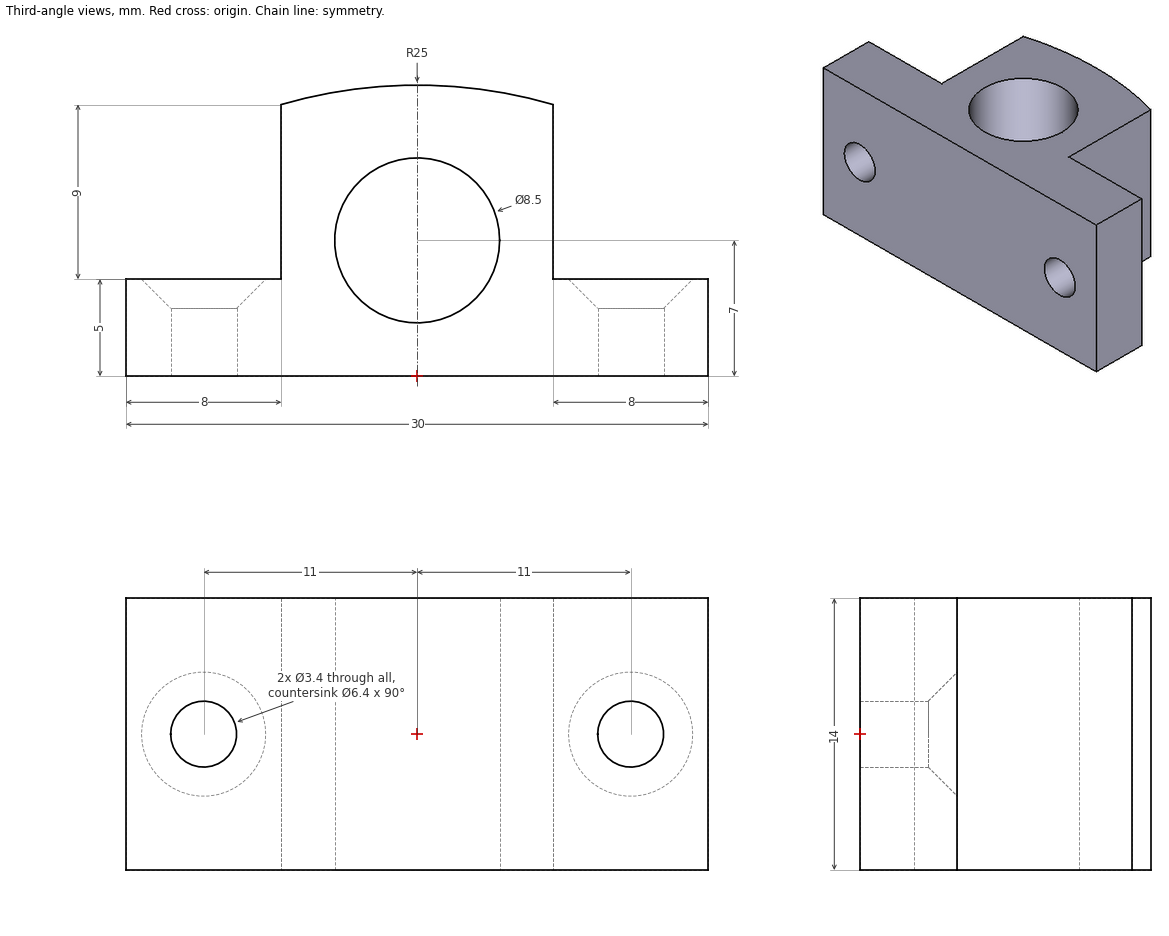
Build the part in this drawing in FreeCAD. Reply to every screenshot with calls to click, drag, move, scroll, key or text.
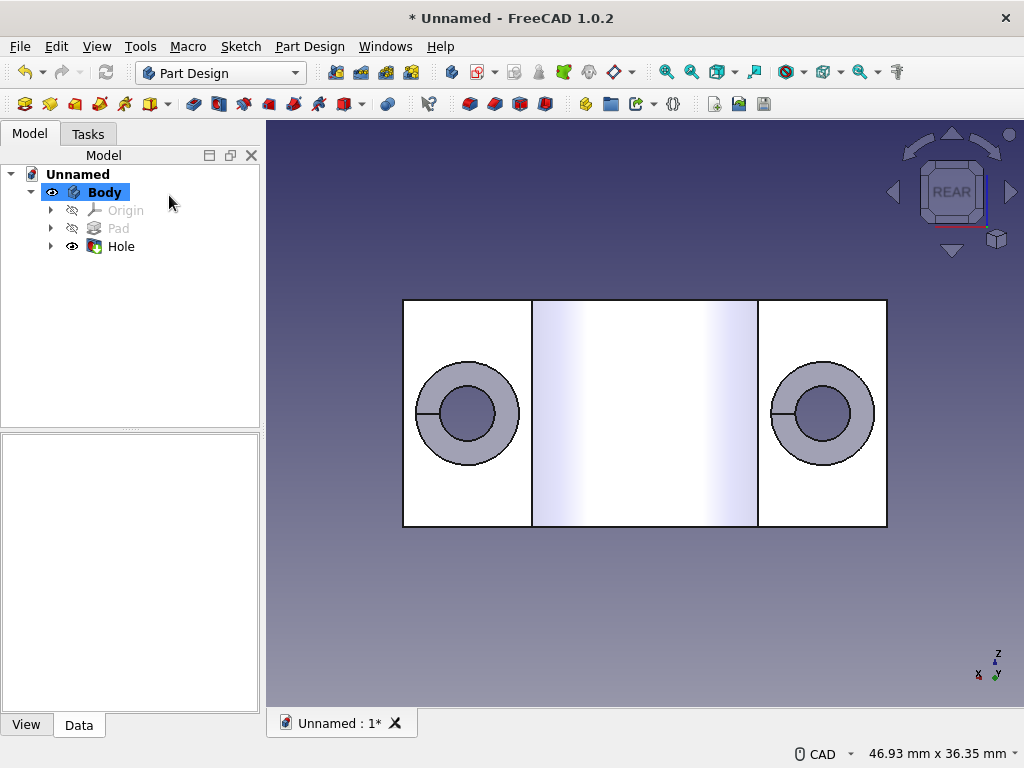
key(0)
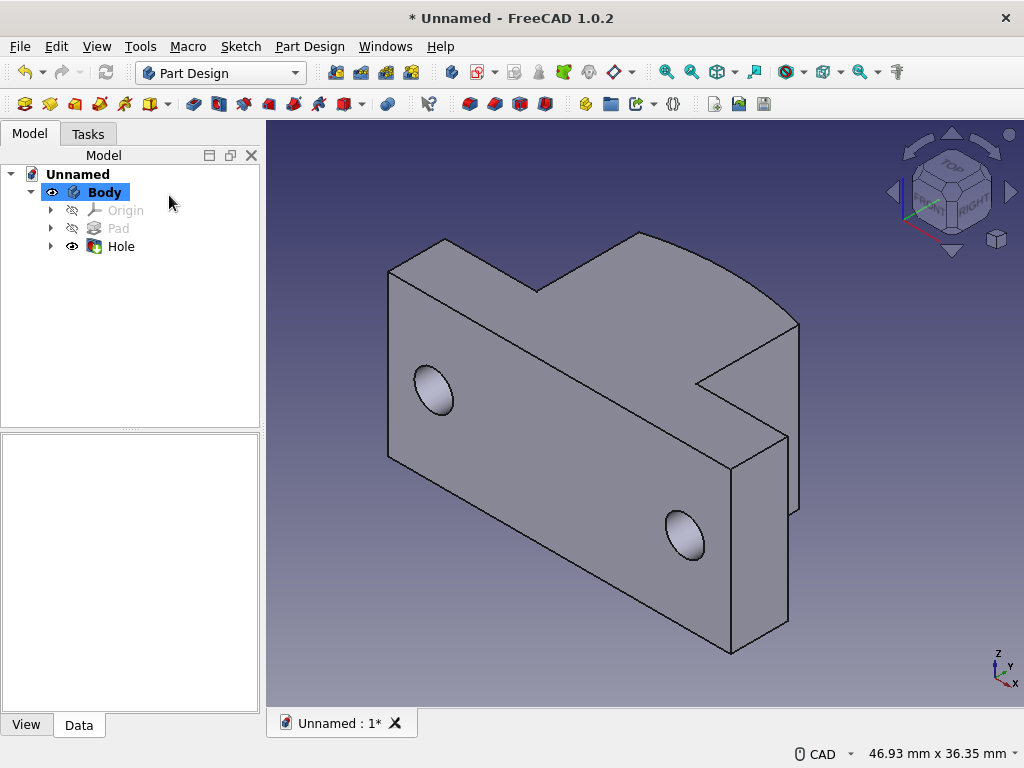
click(645, 320)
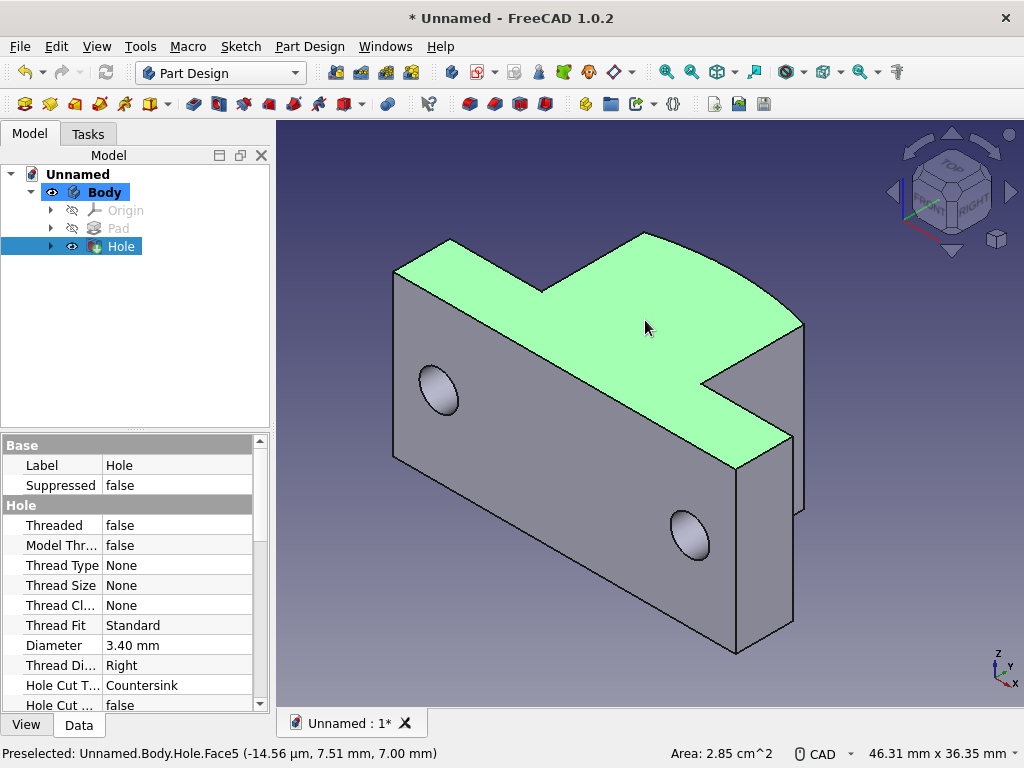
click(476, 72)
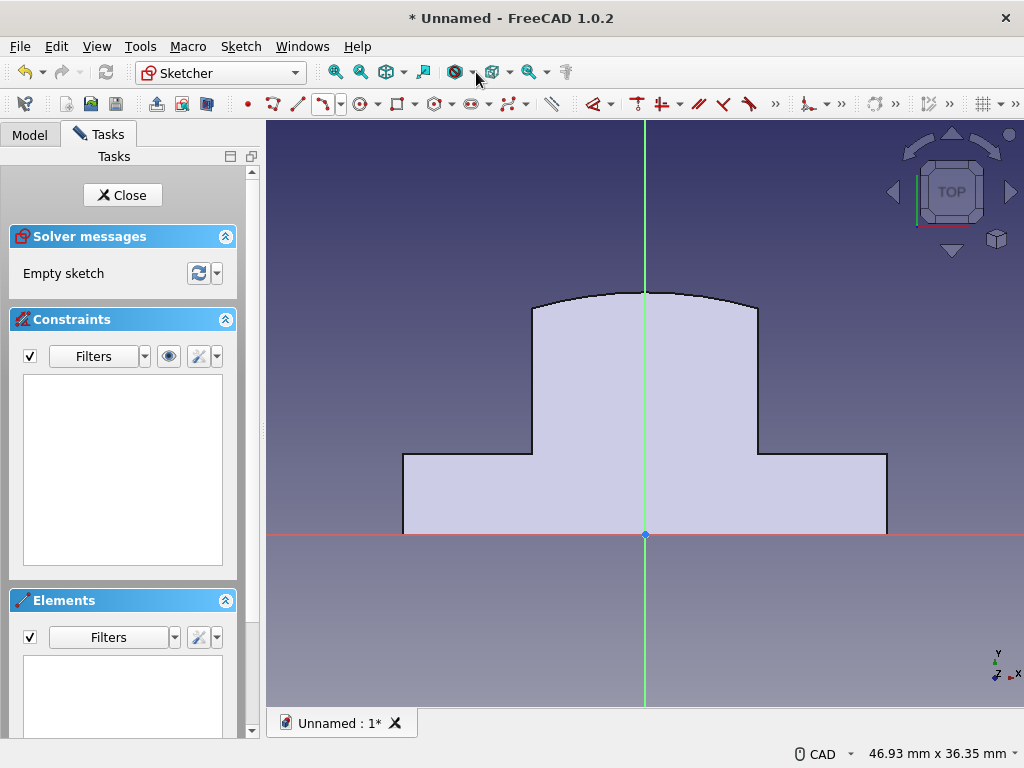
scroll(701, 468, up, 4)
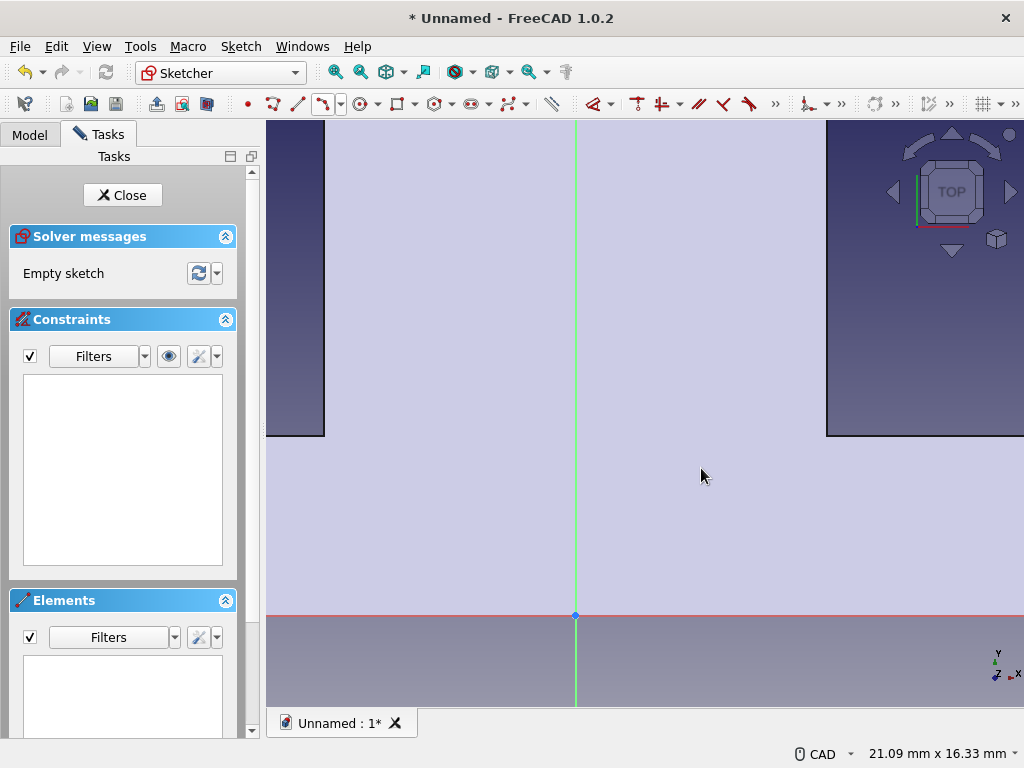
click(360, 104)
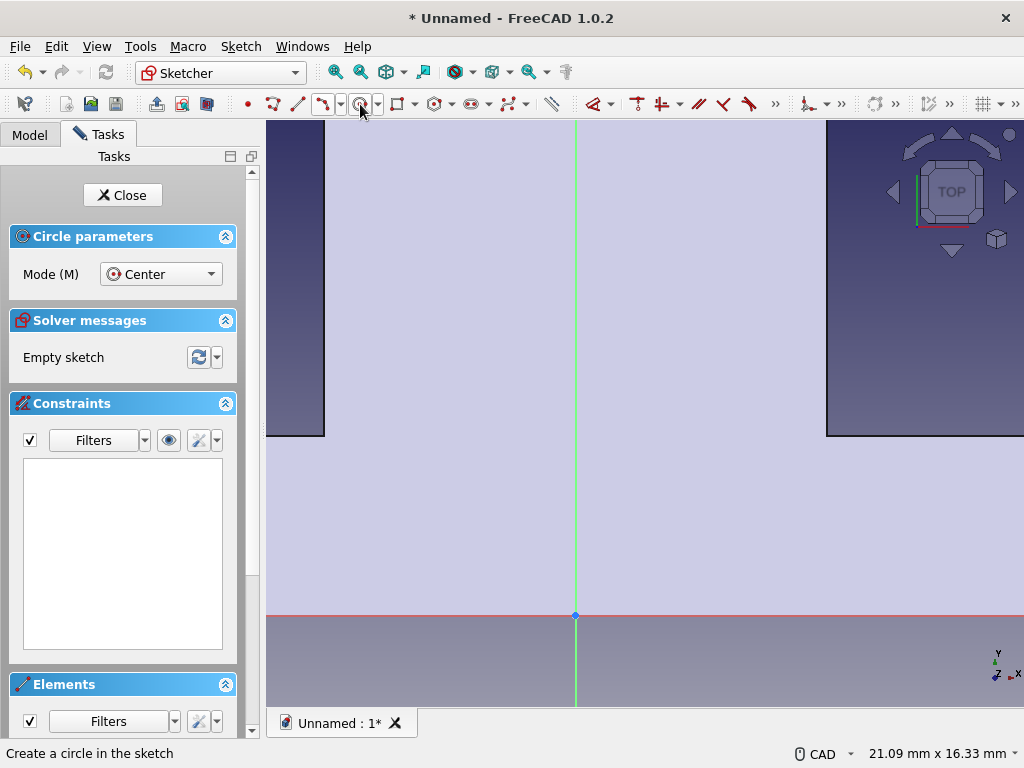
click(576, 364)
move(684, 256)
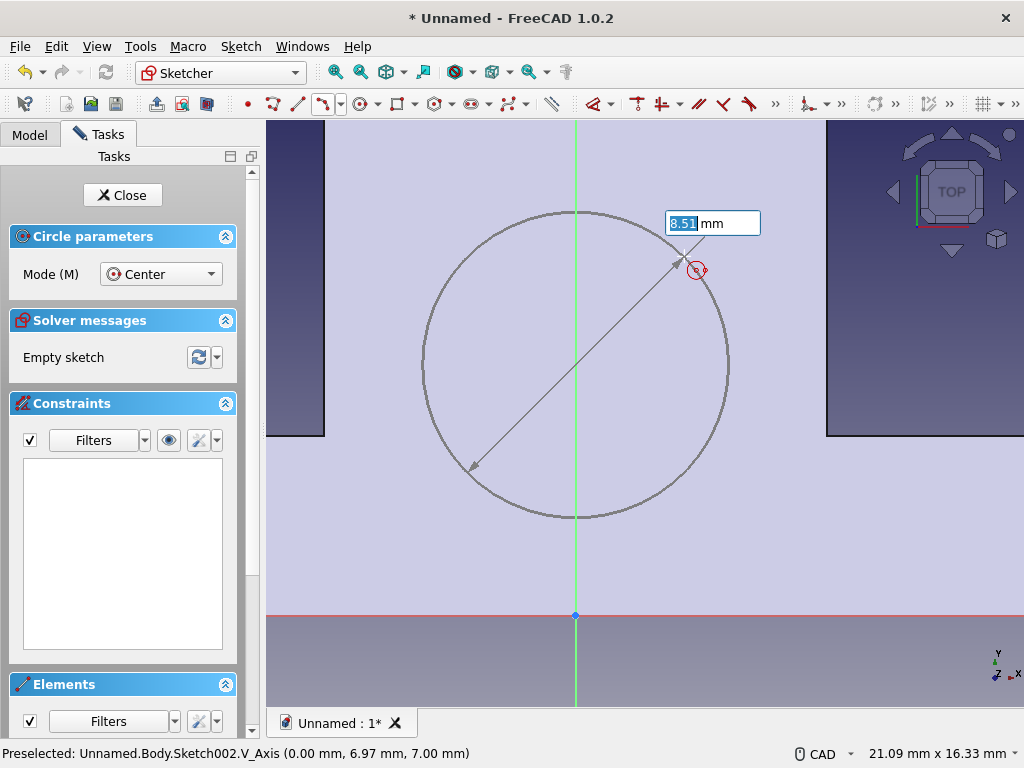
text(8.5)
key(Return)
key(Escape)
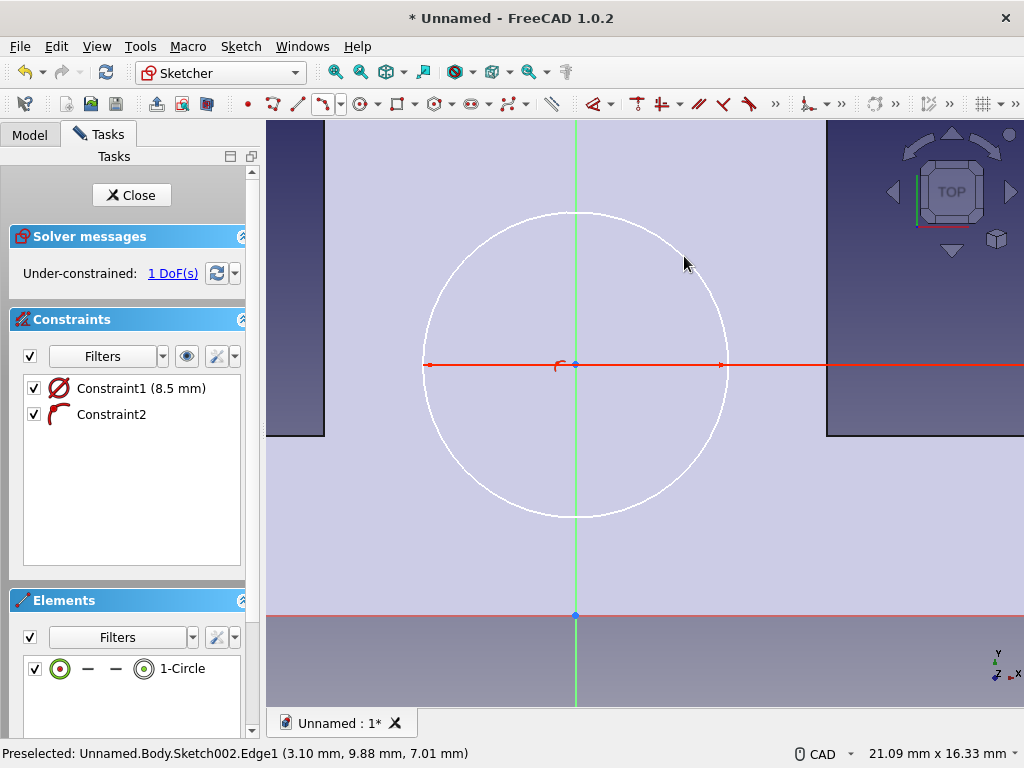
click(592, 104)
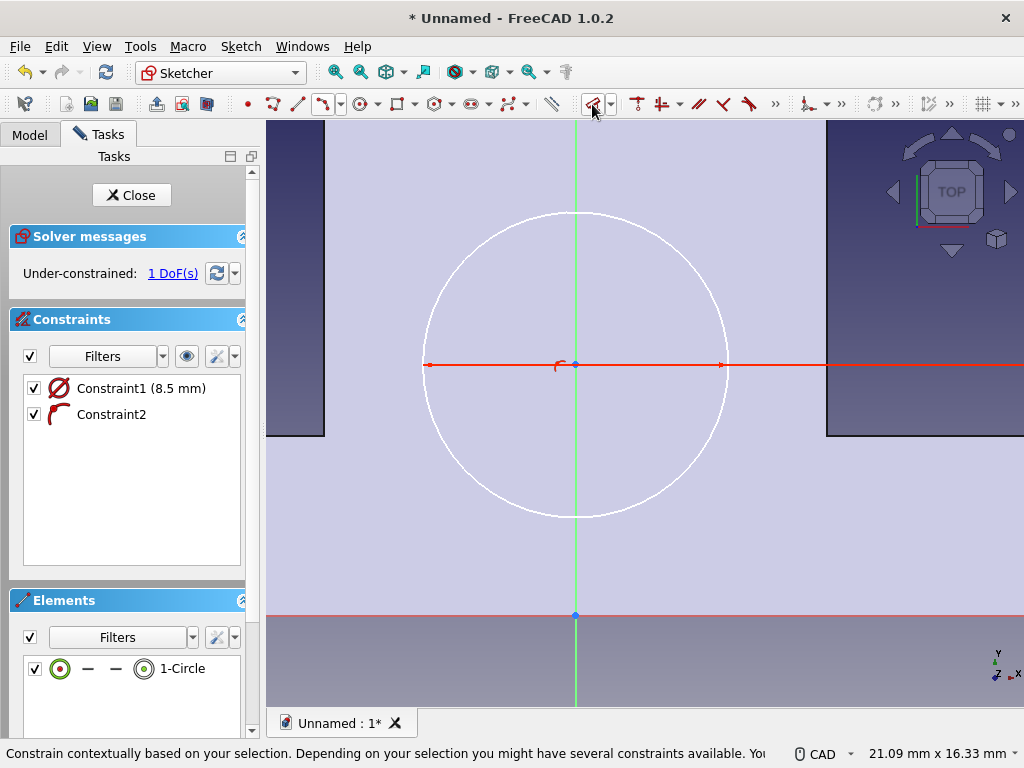
click(576, 365)
click(610, 490)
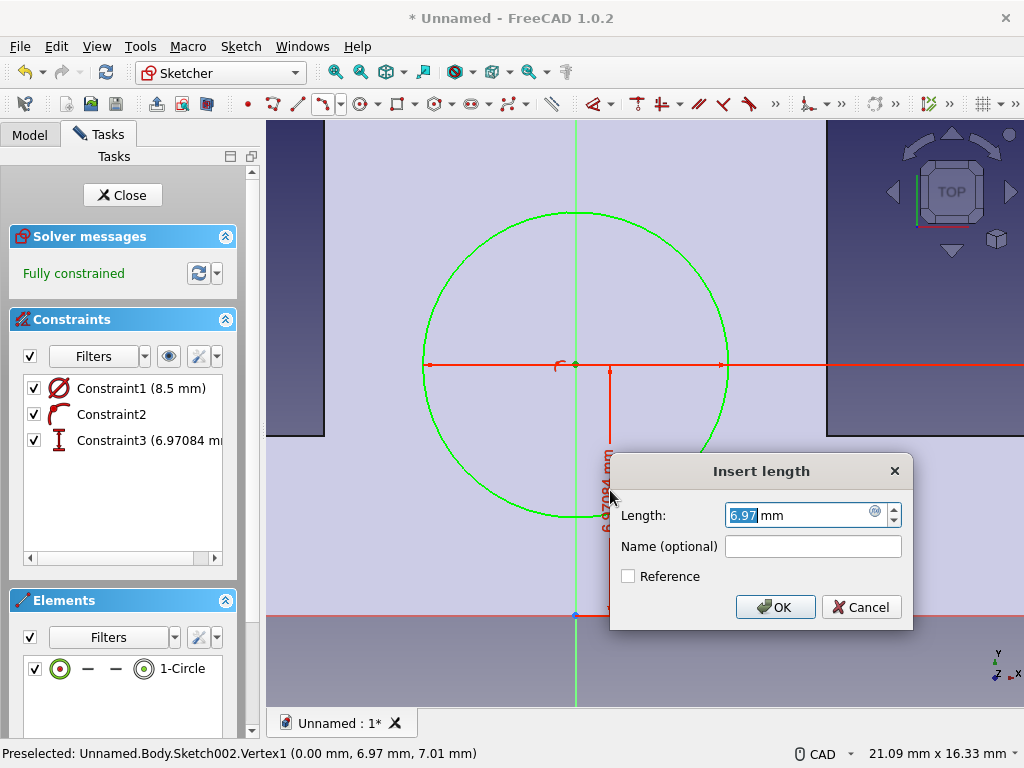
text(7)
key(Return)
key(Escape)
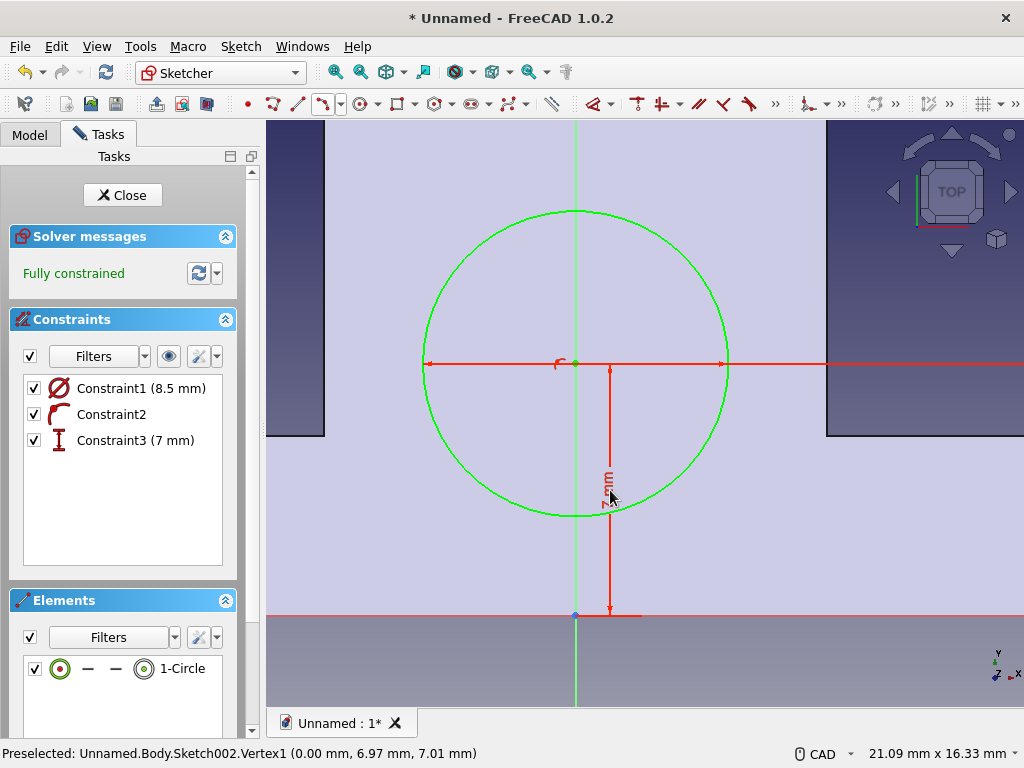
click(123, 195)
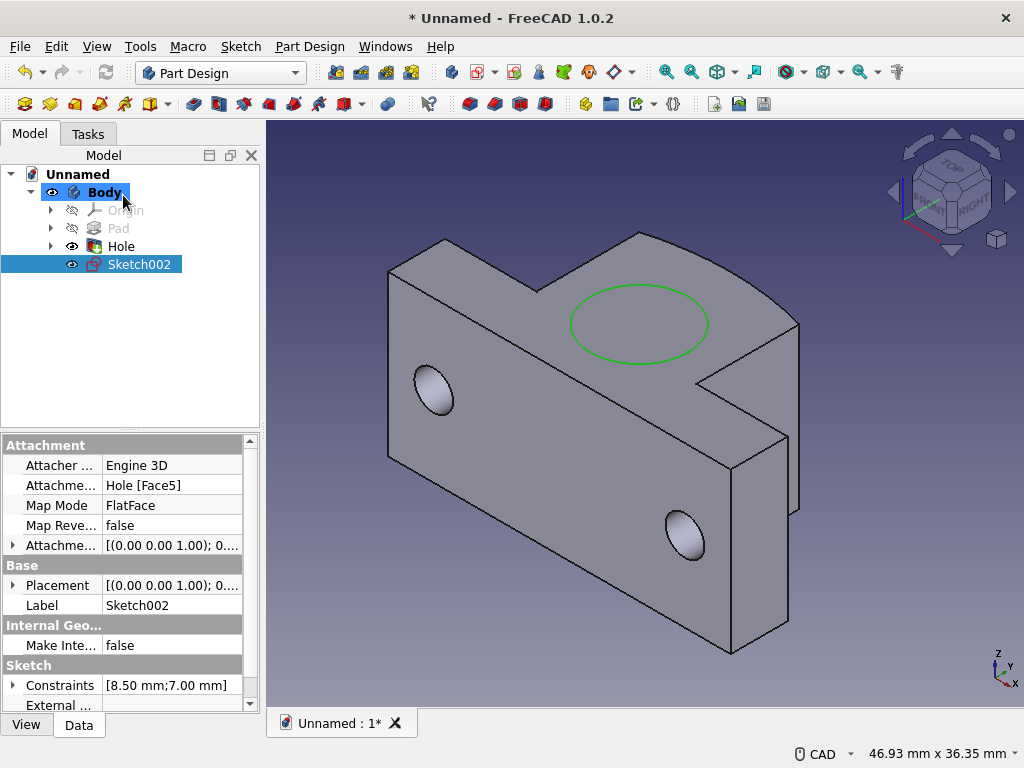
click(194, 104)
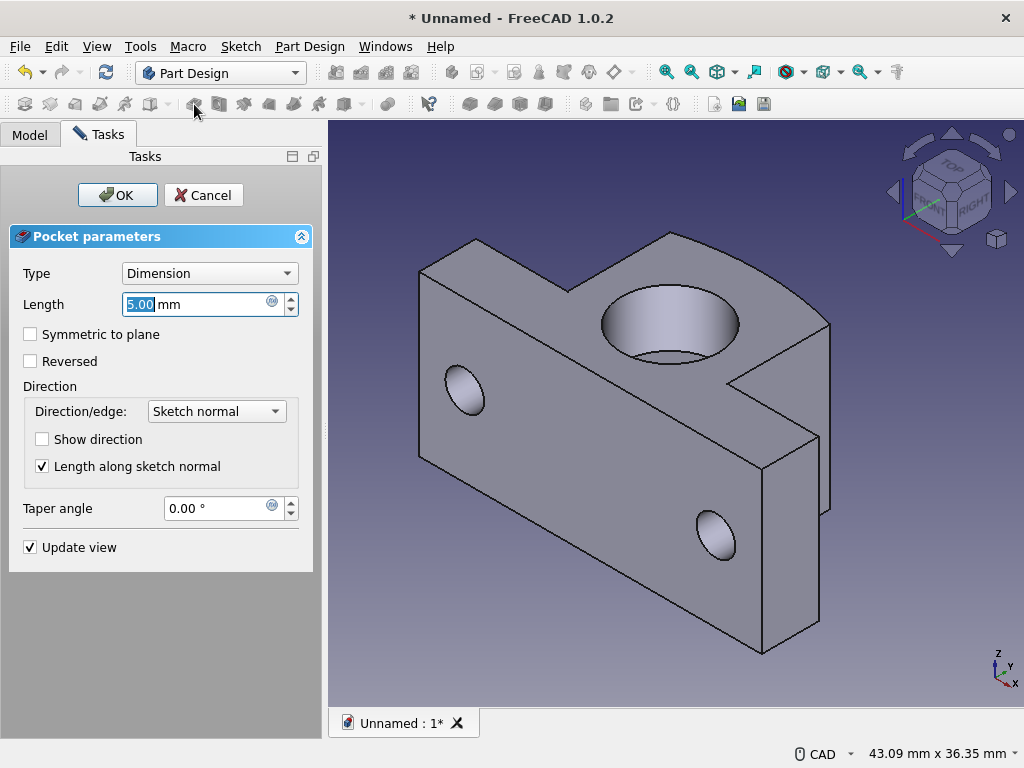
click(210, 274)